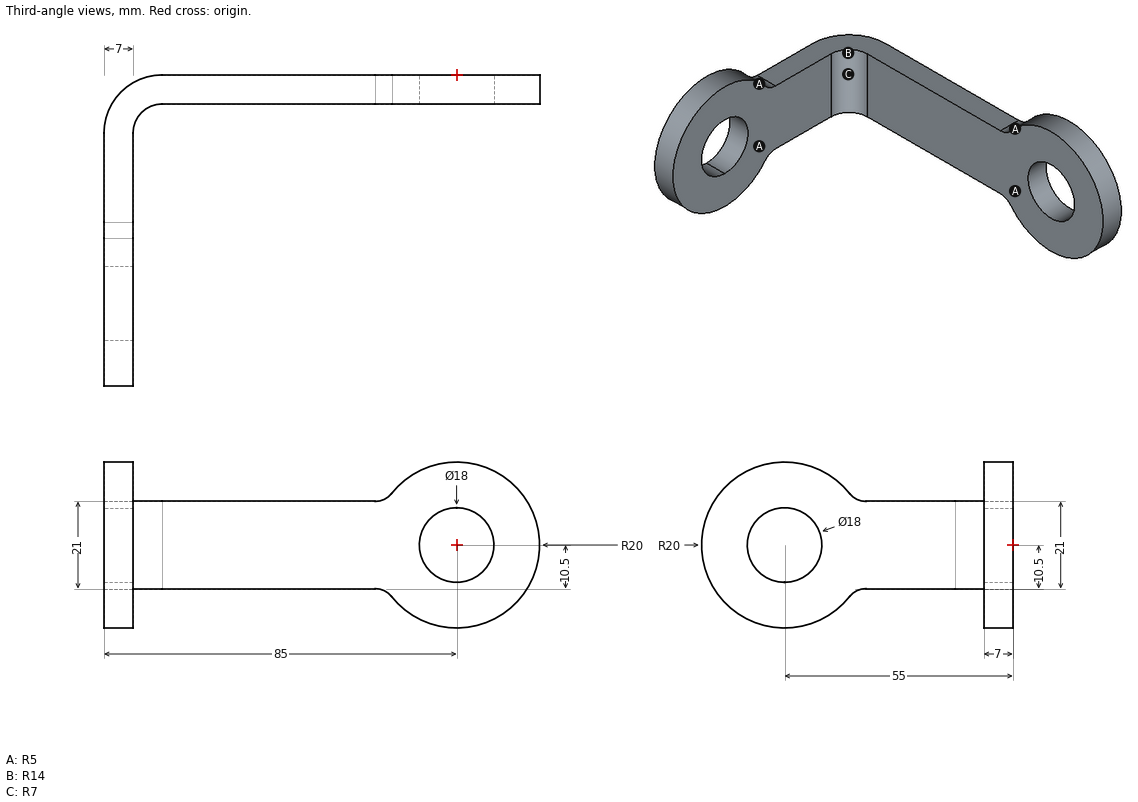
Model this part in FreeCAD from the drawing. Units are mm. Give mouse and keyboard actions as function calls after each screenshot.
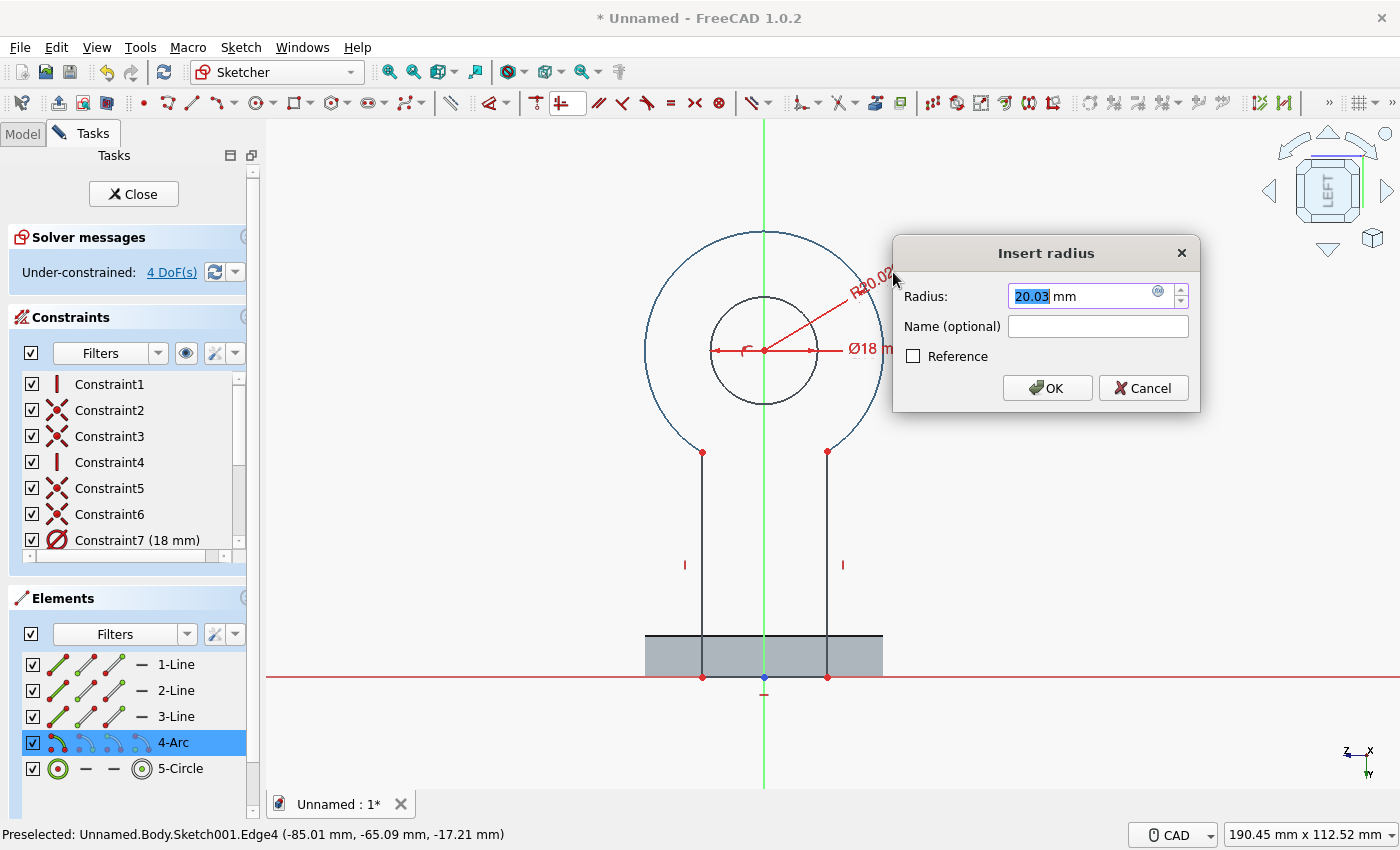
text(20)
key(Return)
key(Escape)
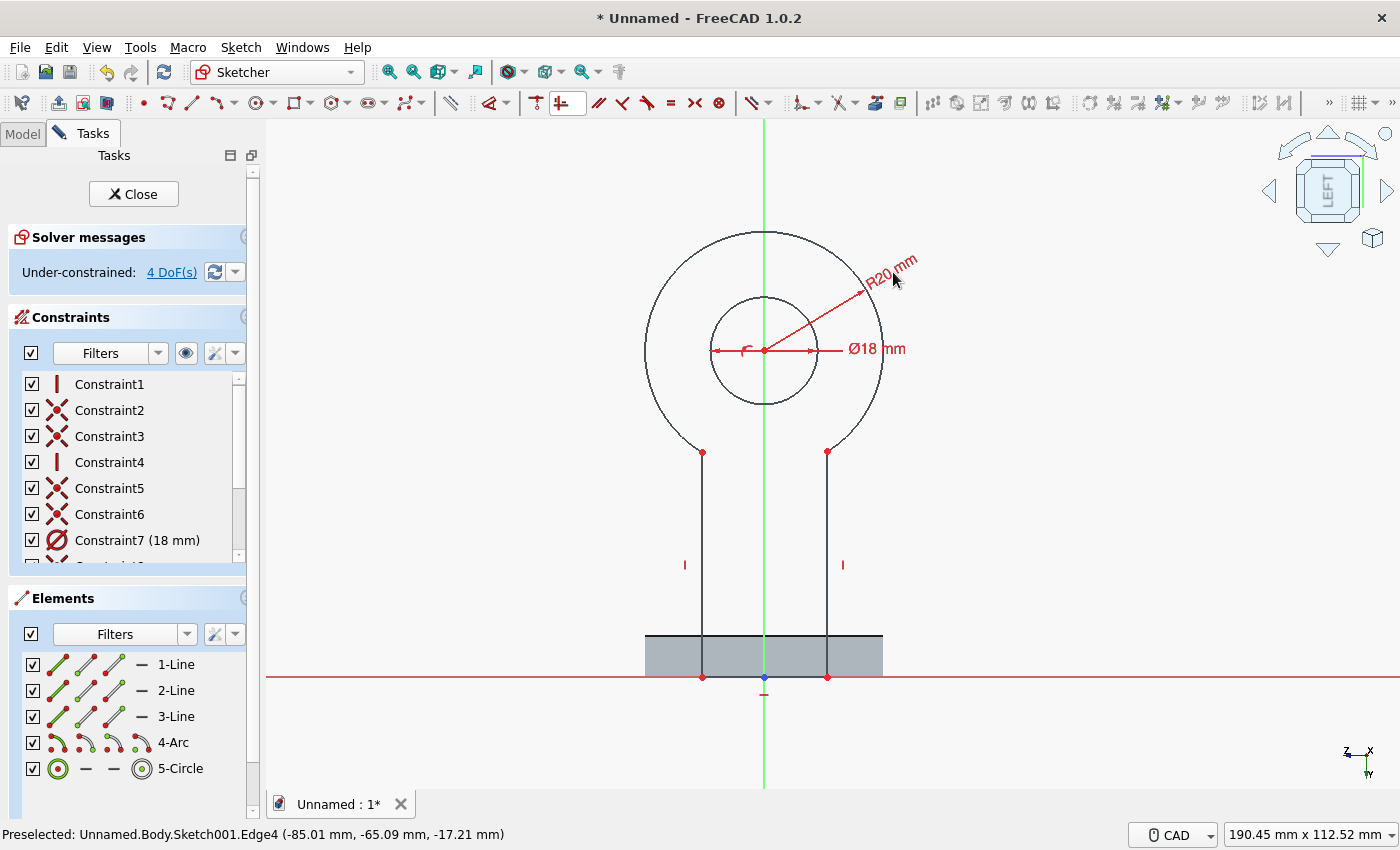
click(827, 677)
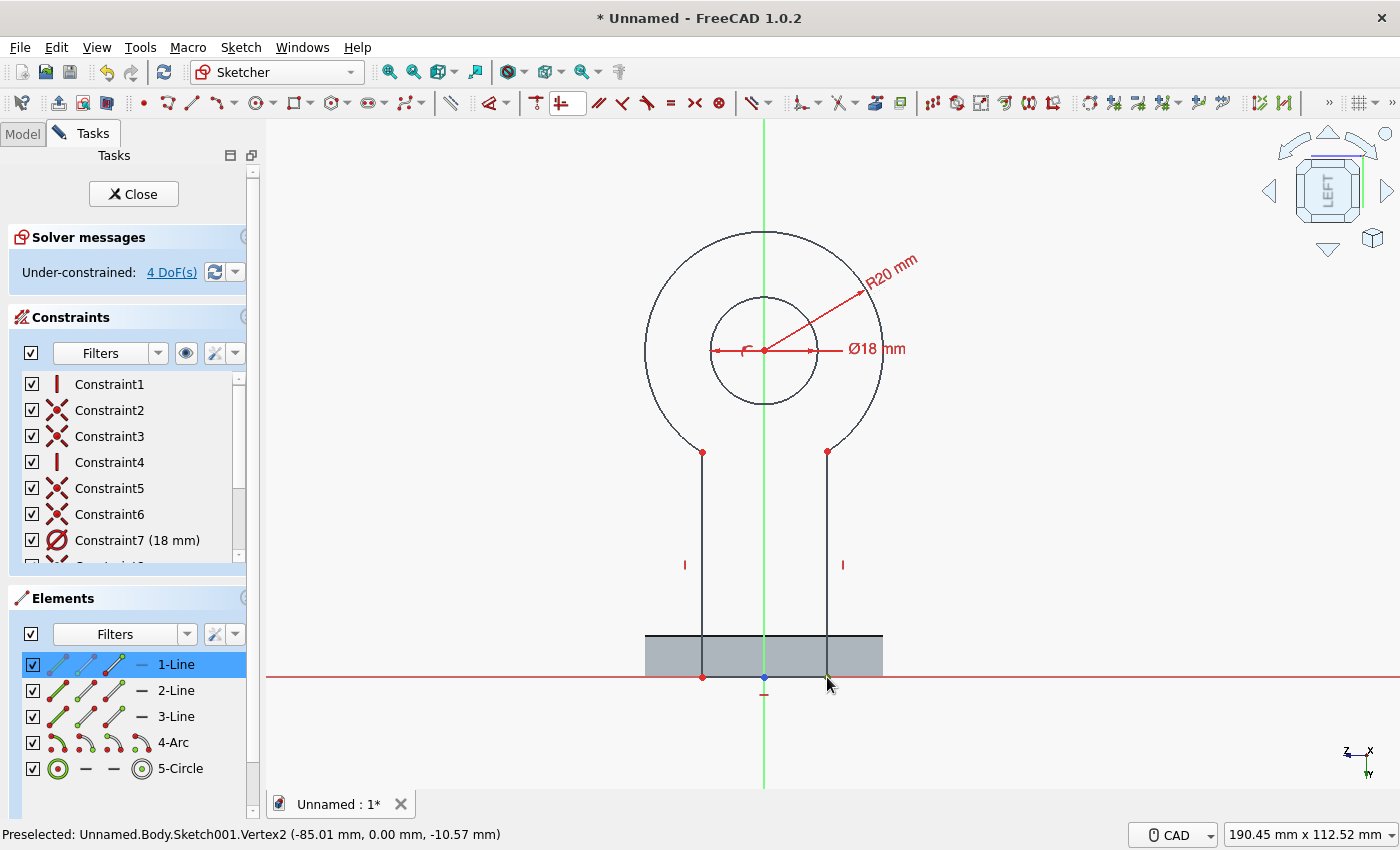
click(361, 677)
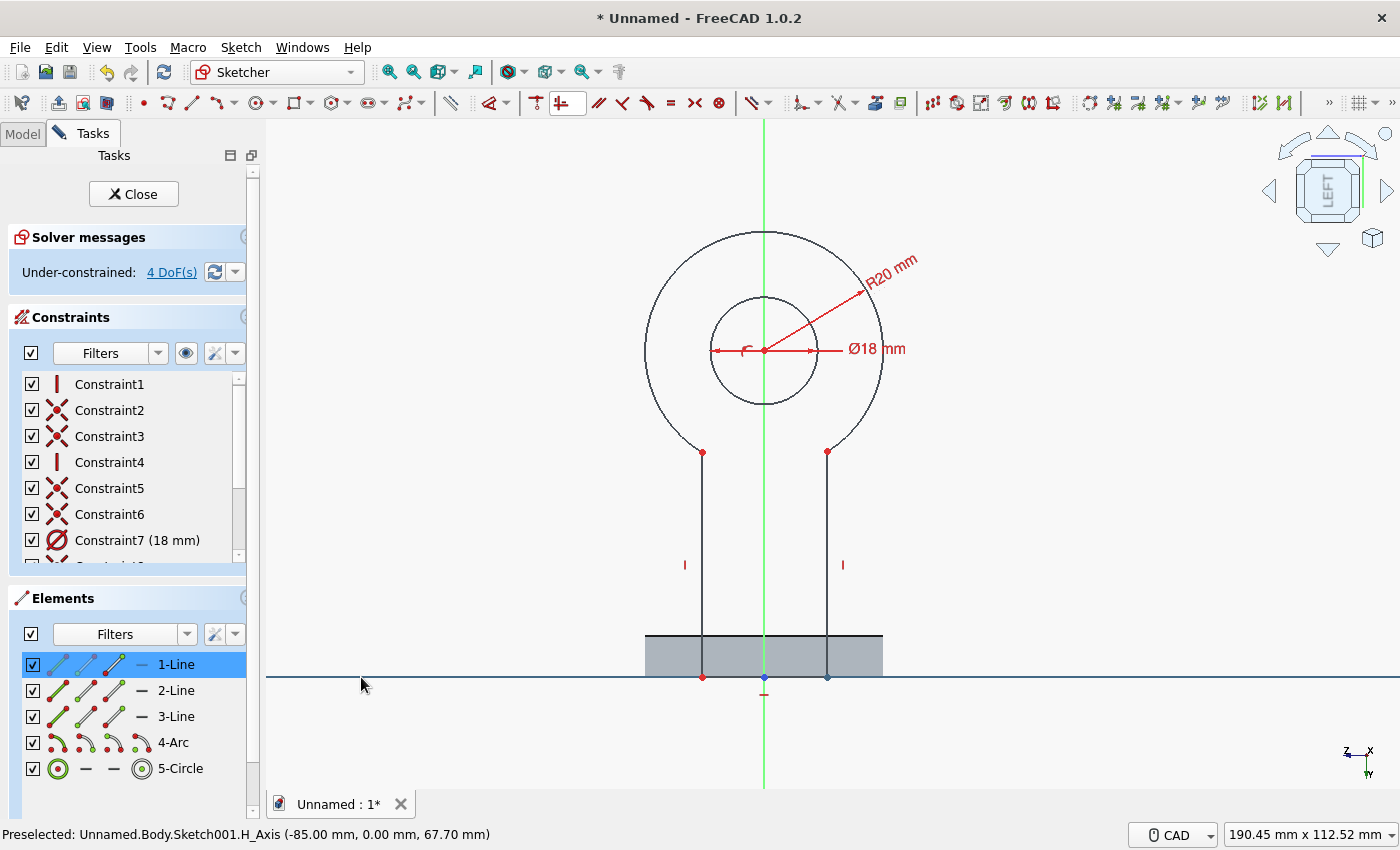
click(536, 104)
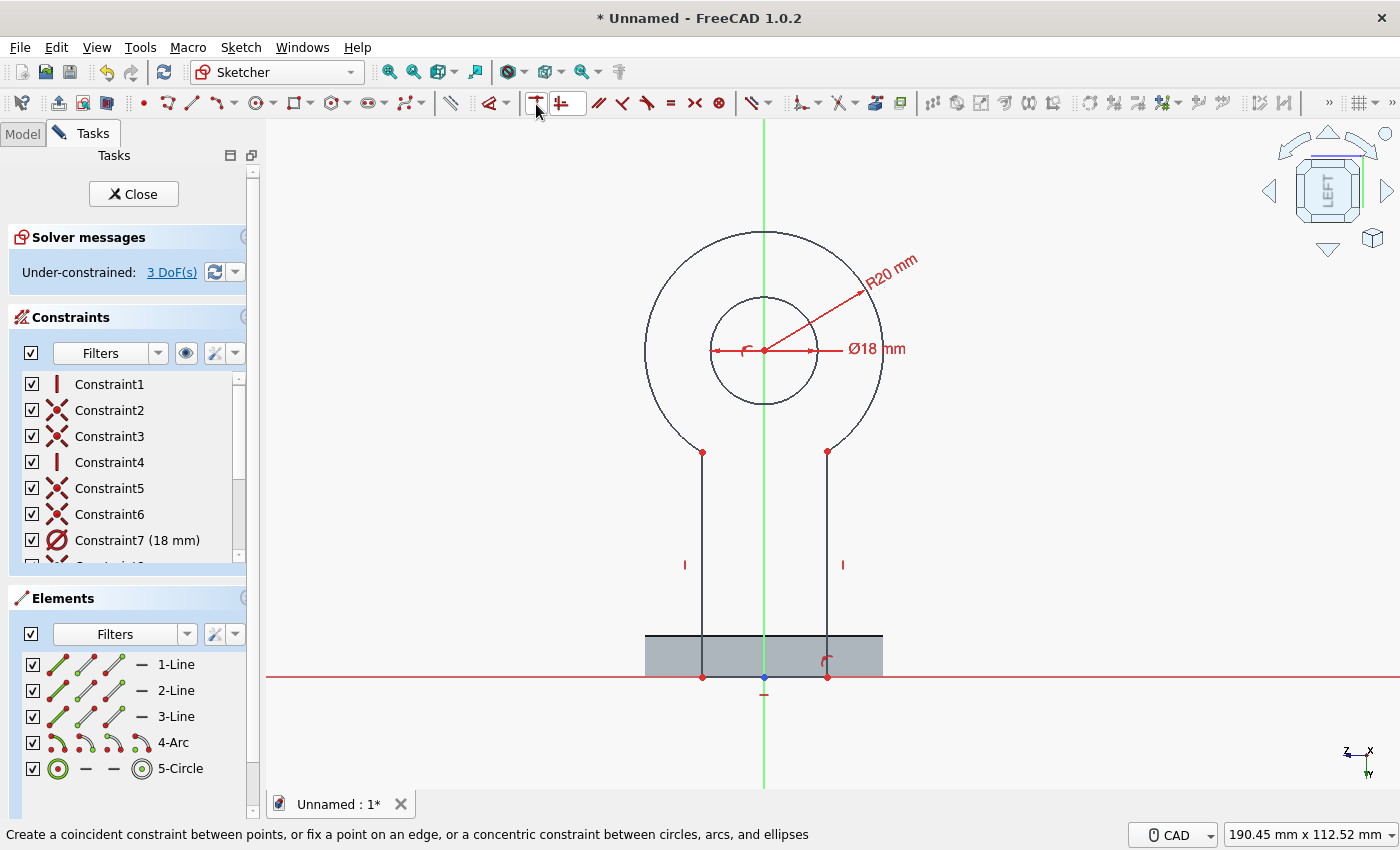
click(490, 104)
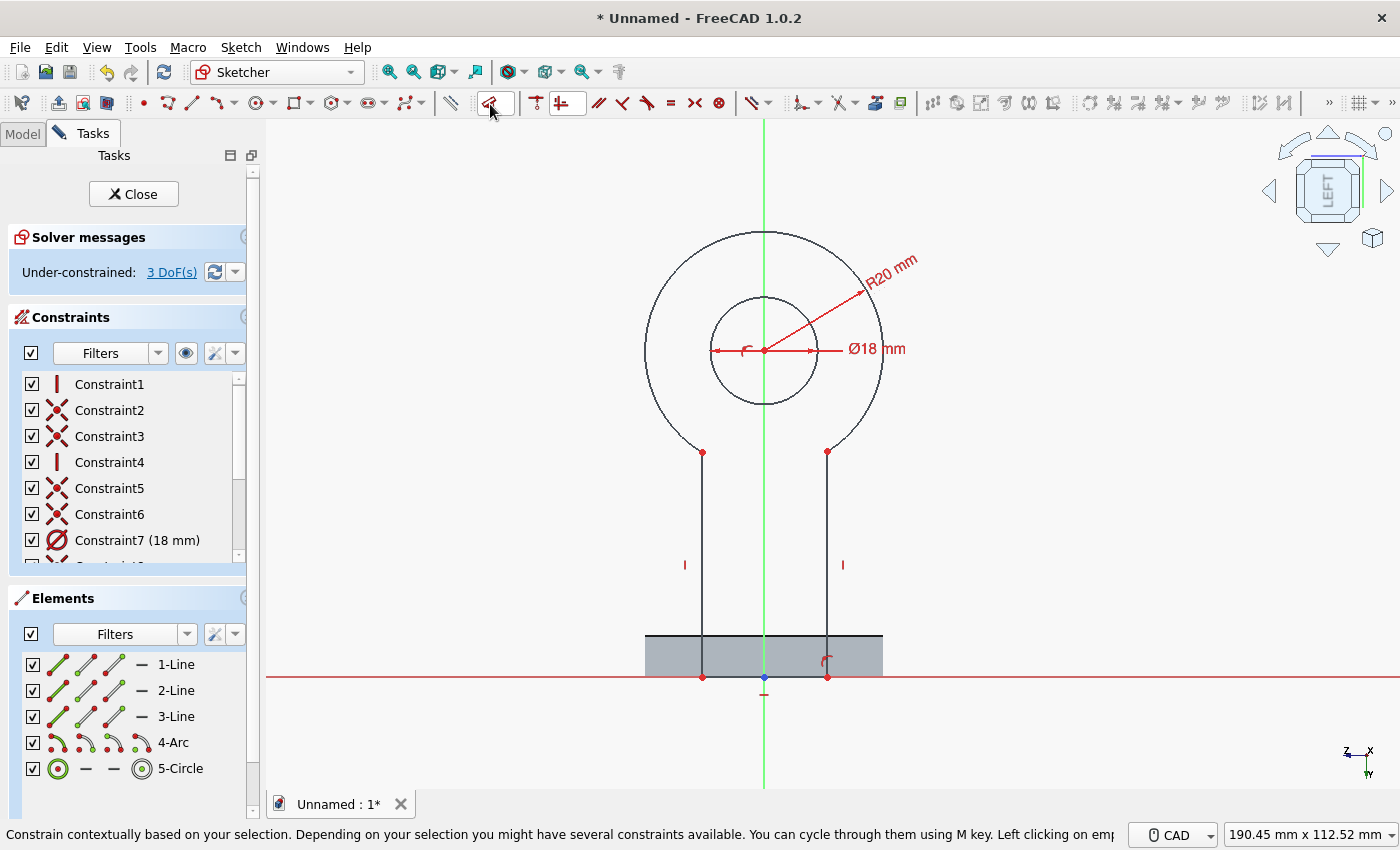
click(790, 677)
click(736, 711)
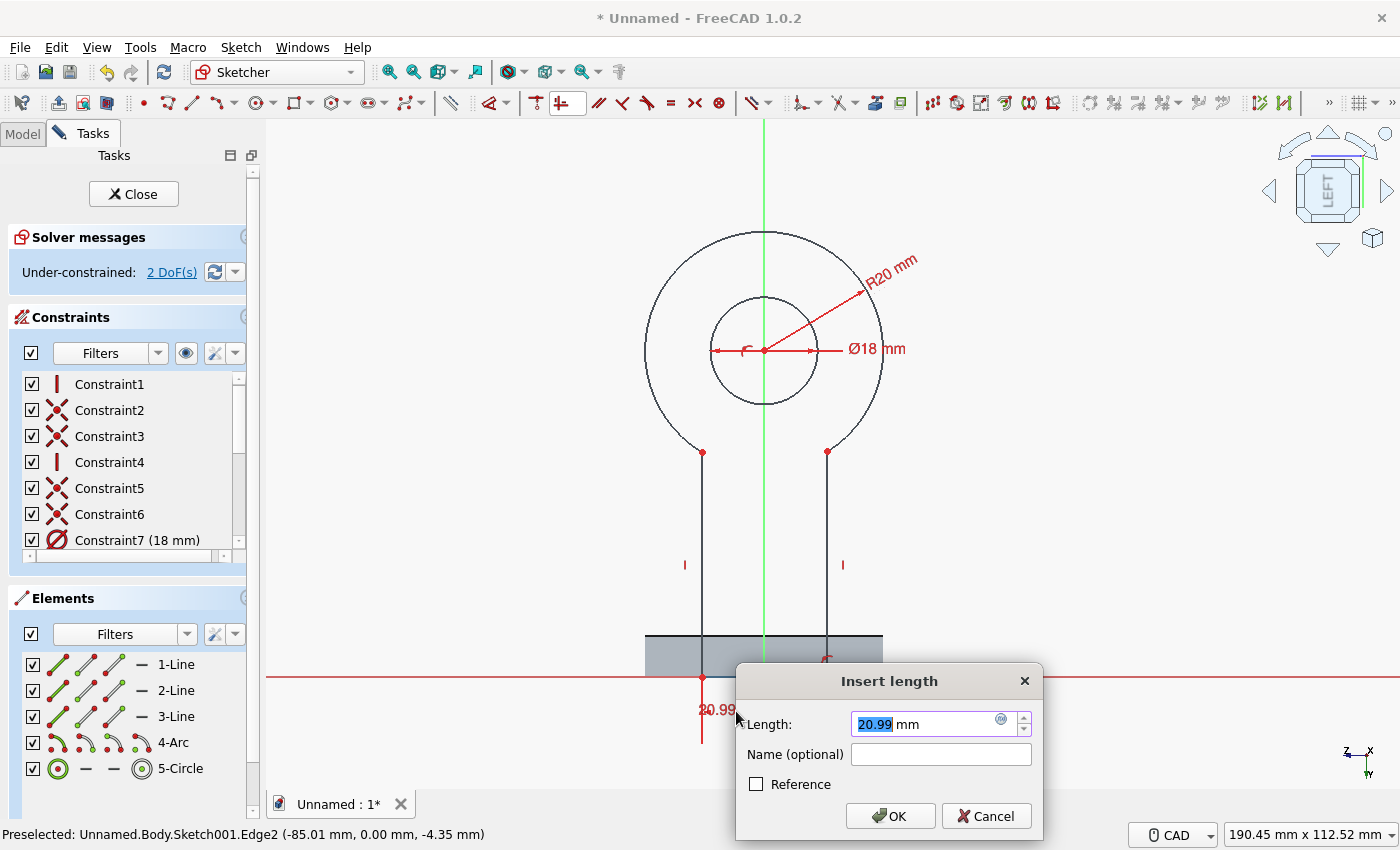
text(21)
key(Return)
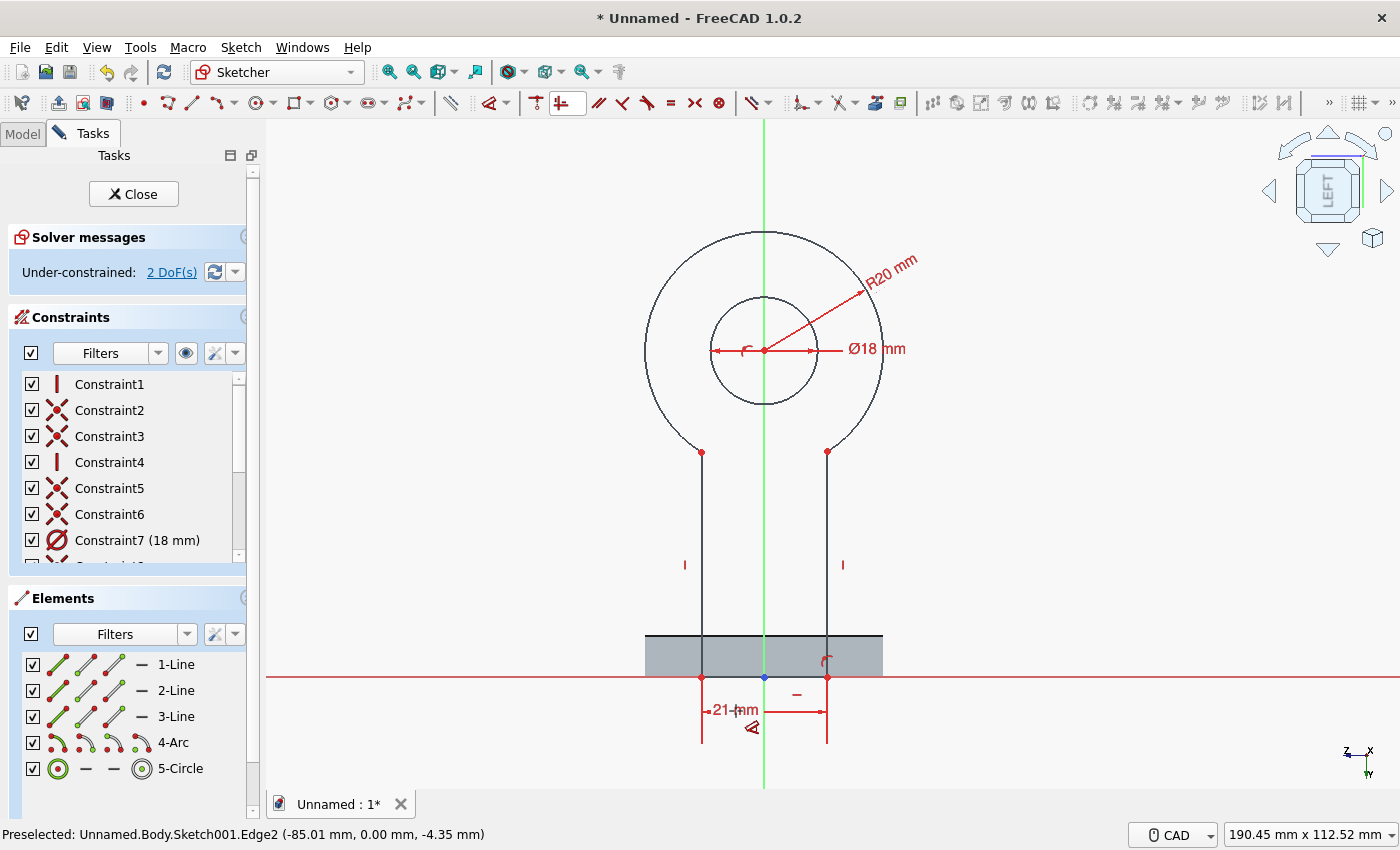
click(764, 351)
click(798, 514)